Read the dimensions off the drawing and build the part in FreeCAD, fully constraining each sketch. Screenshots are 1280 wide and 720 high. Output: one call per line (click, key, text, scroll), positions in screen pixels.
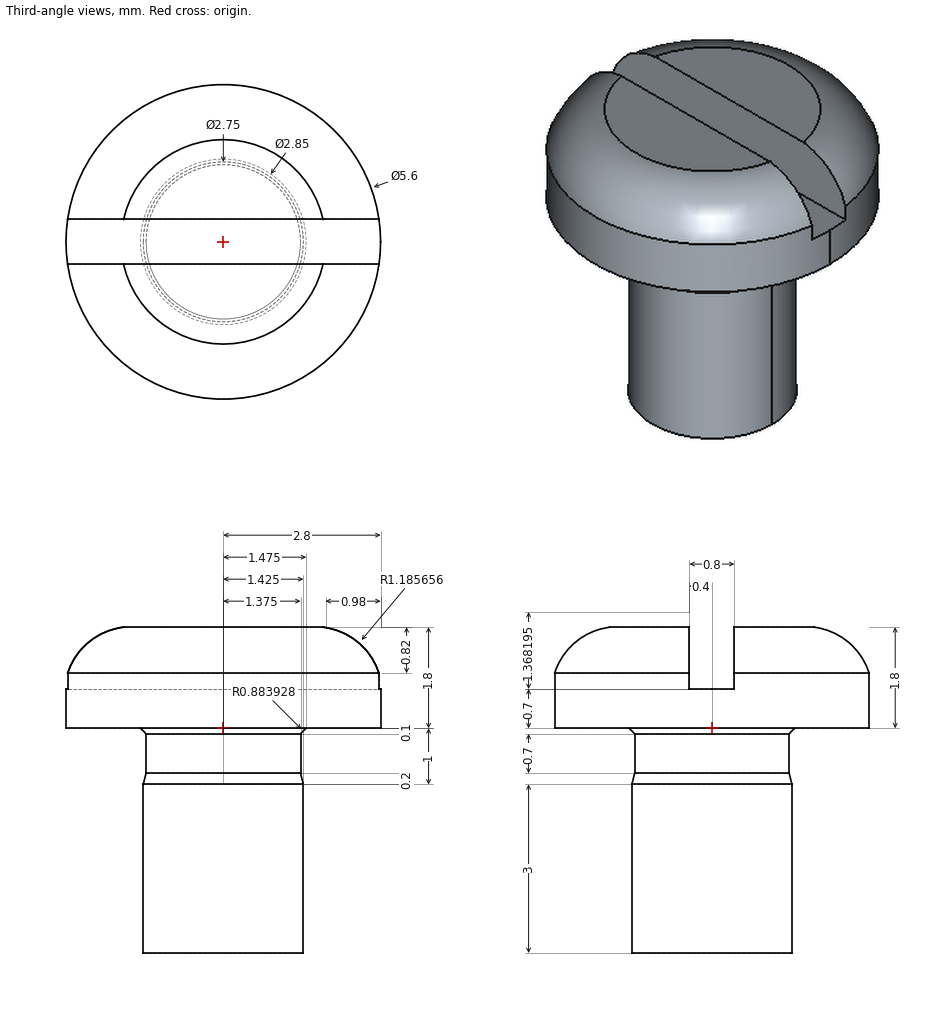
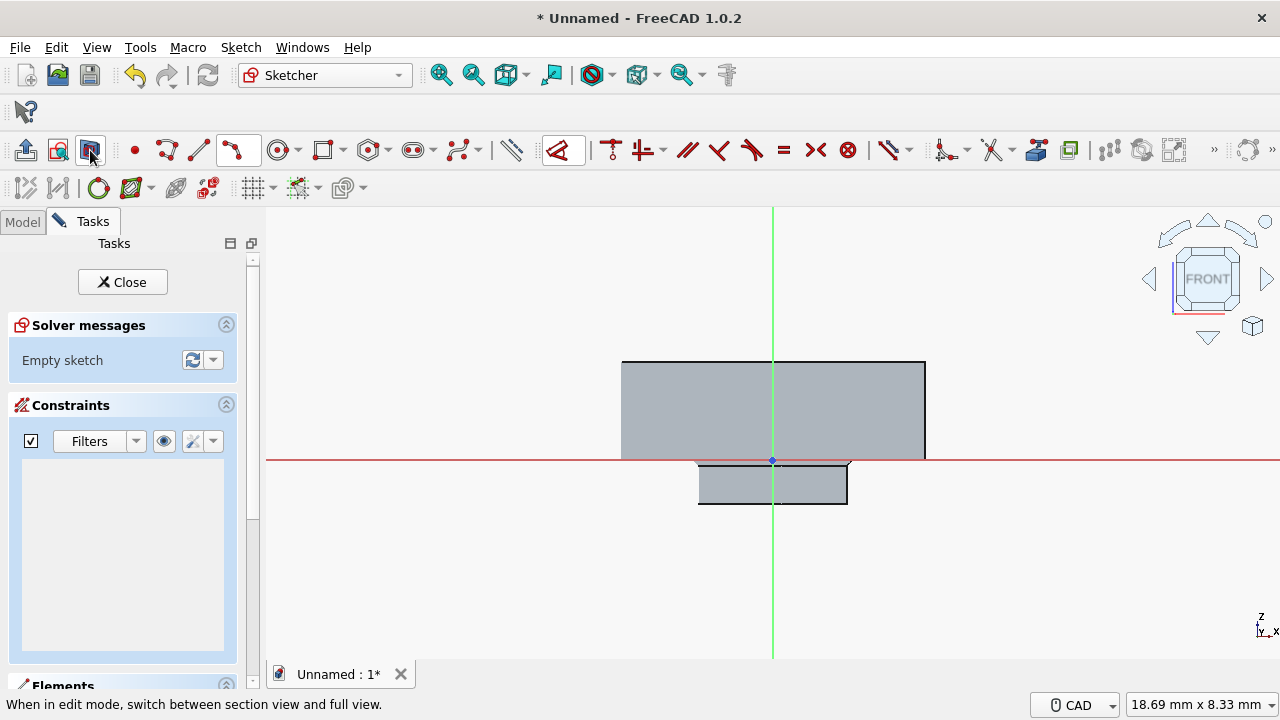
scroll(839, 501, up, 8)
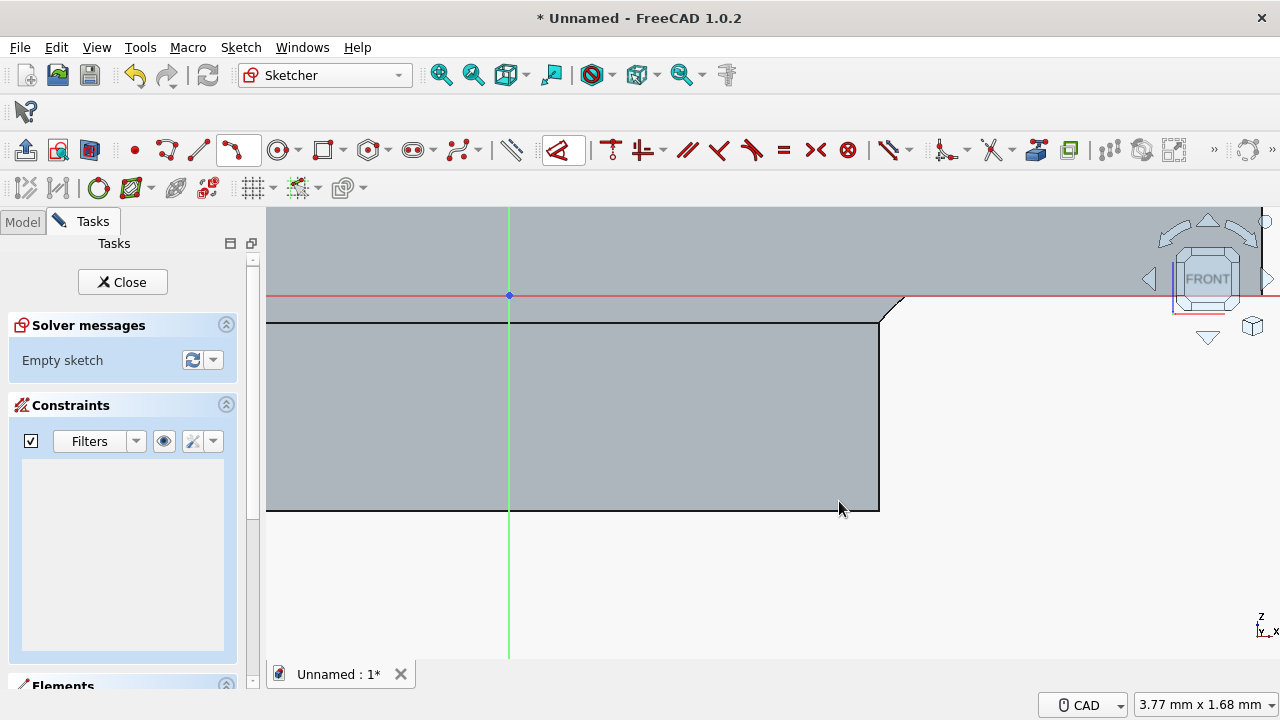
click(168, 150)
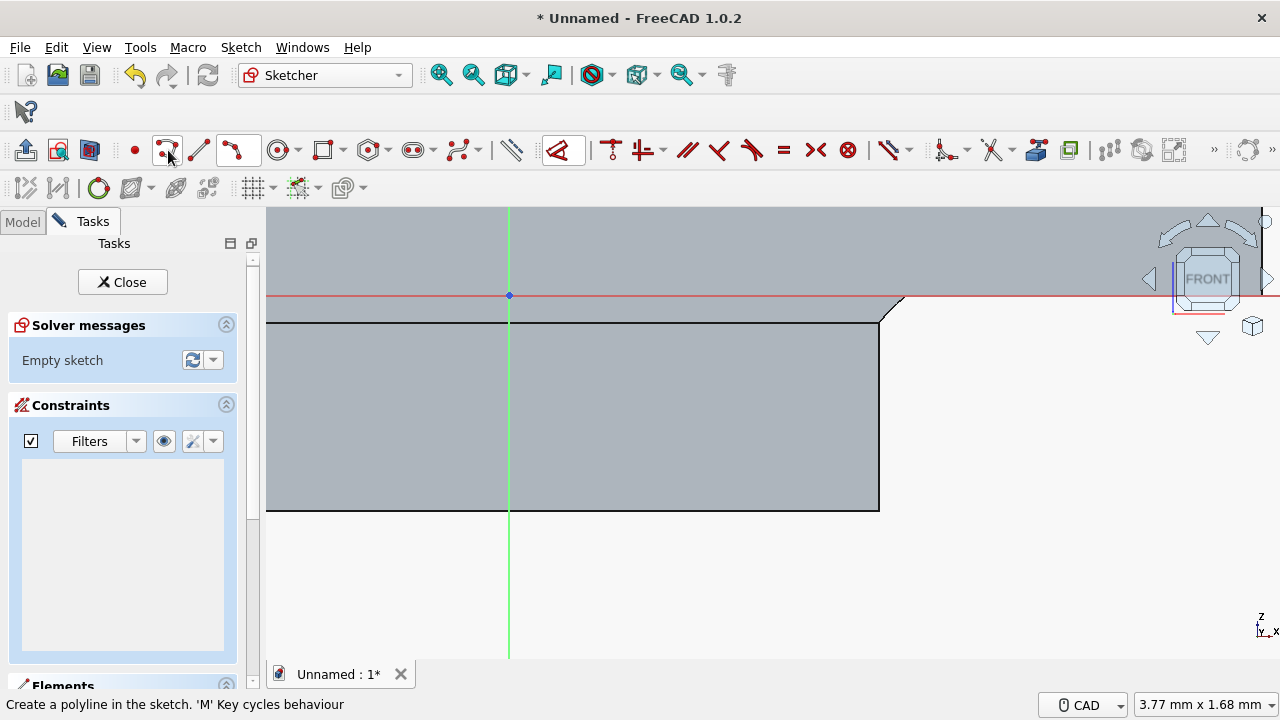
click(509, 511)
click(879, 511)
click(892, 565)
click(518, 565)
click(509, 512)
key(Escape)
key(Escape)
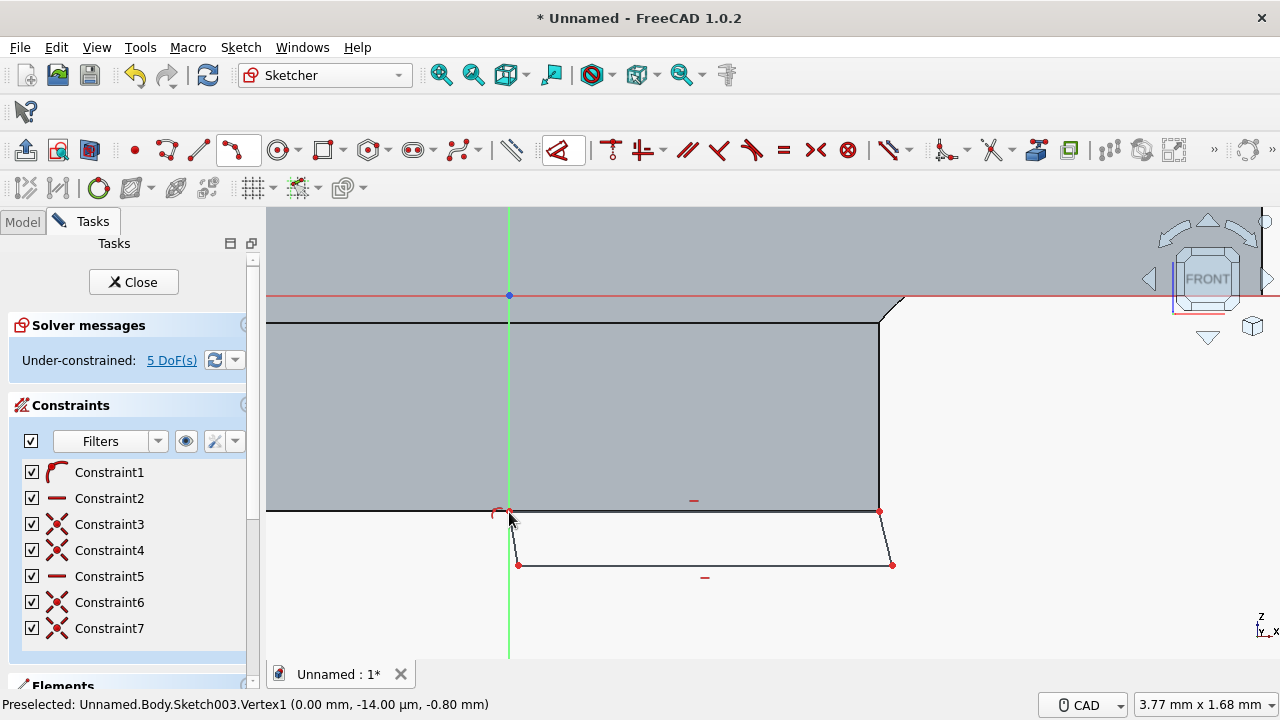
click(512, 528)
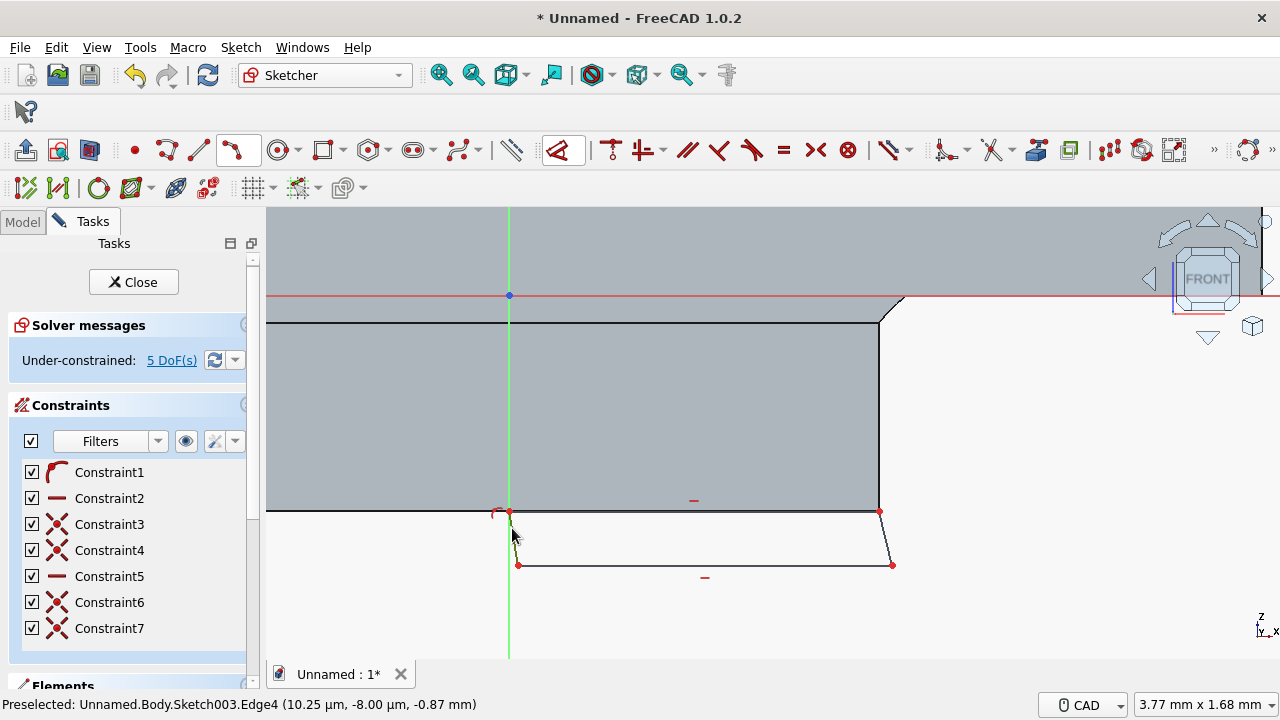
click(666, 150)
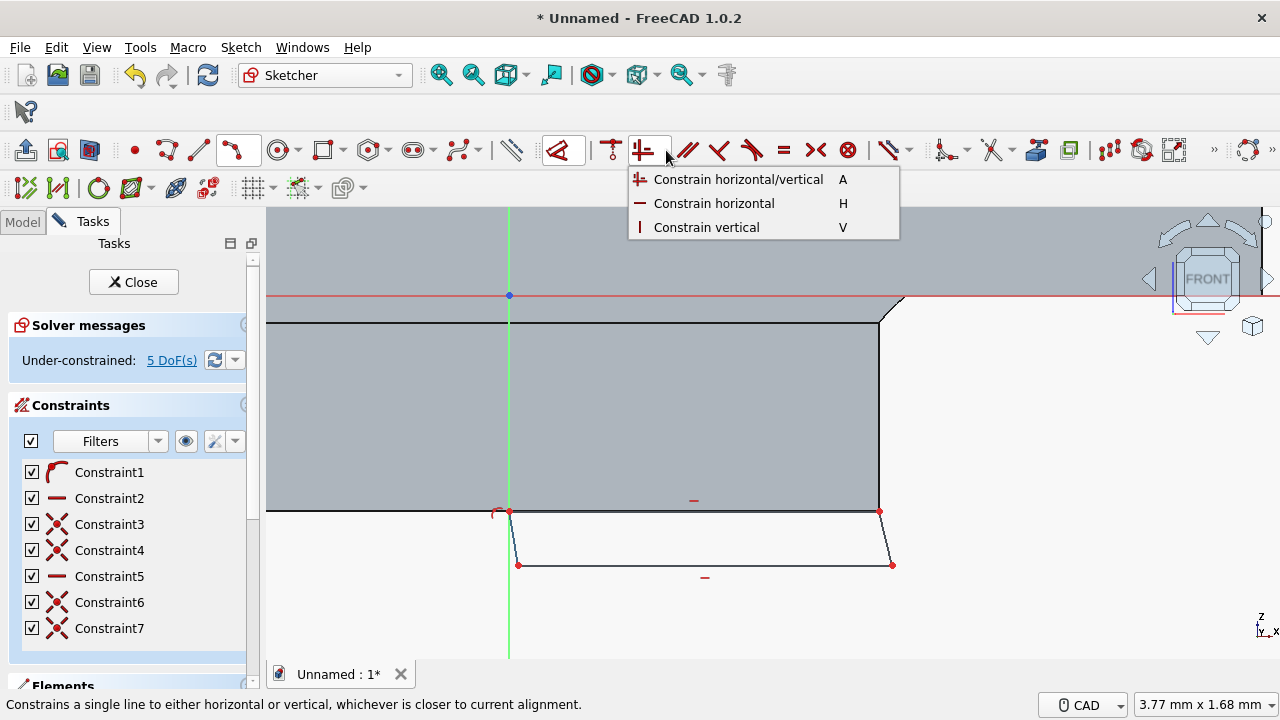
click(764, 227)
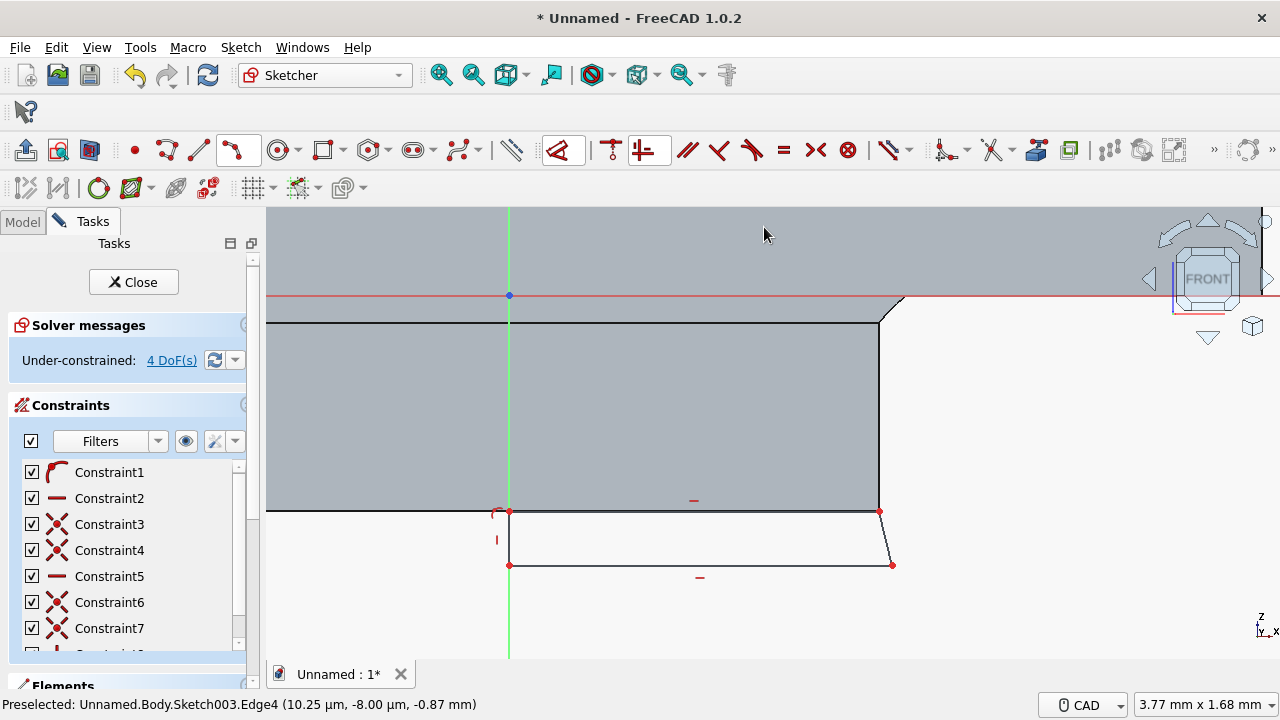
click(892, 566)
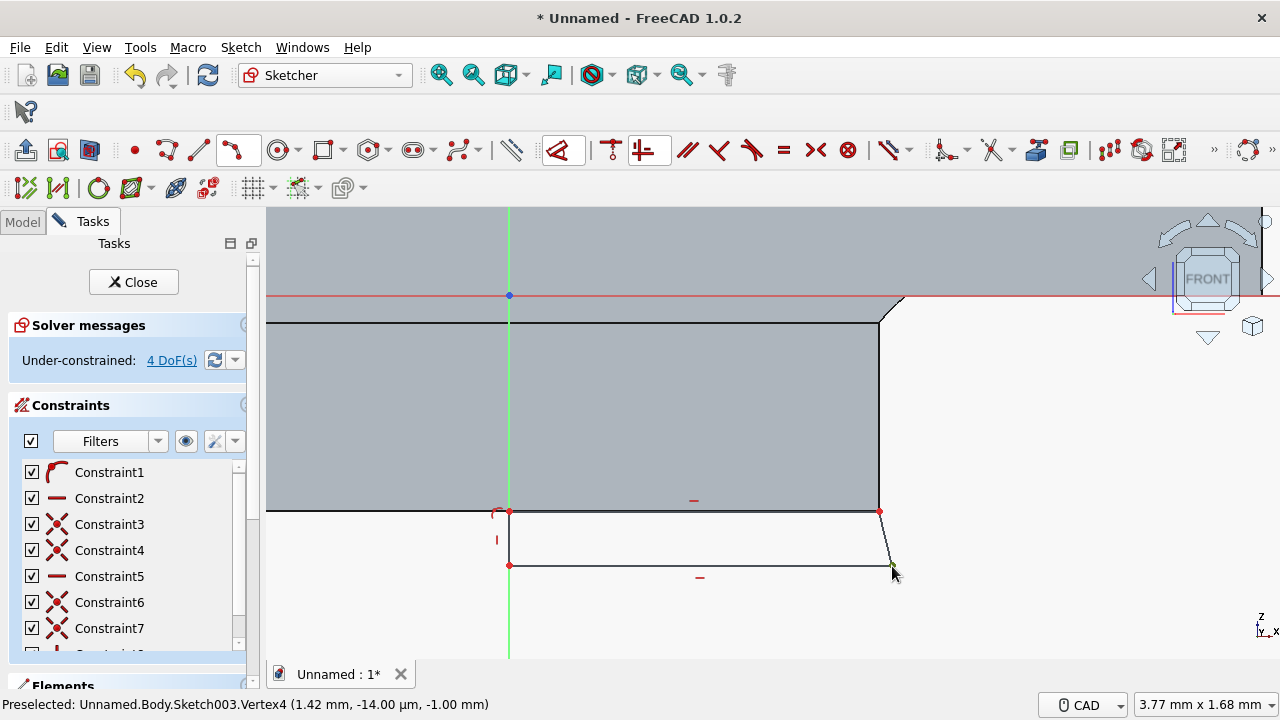
click(580, 150)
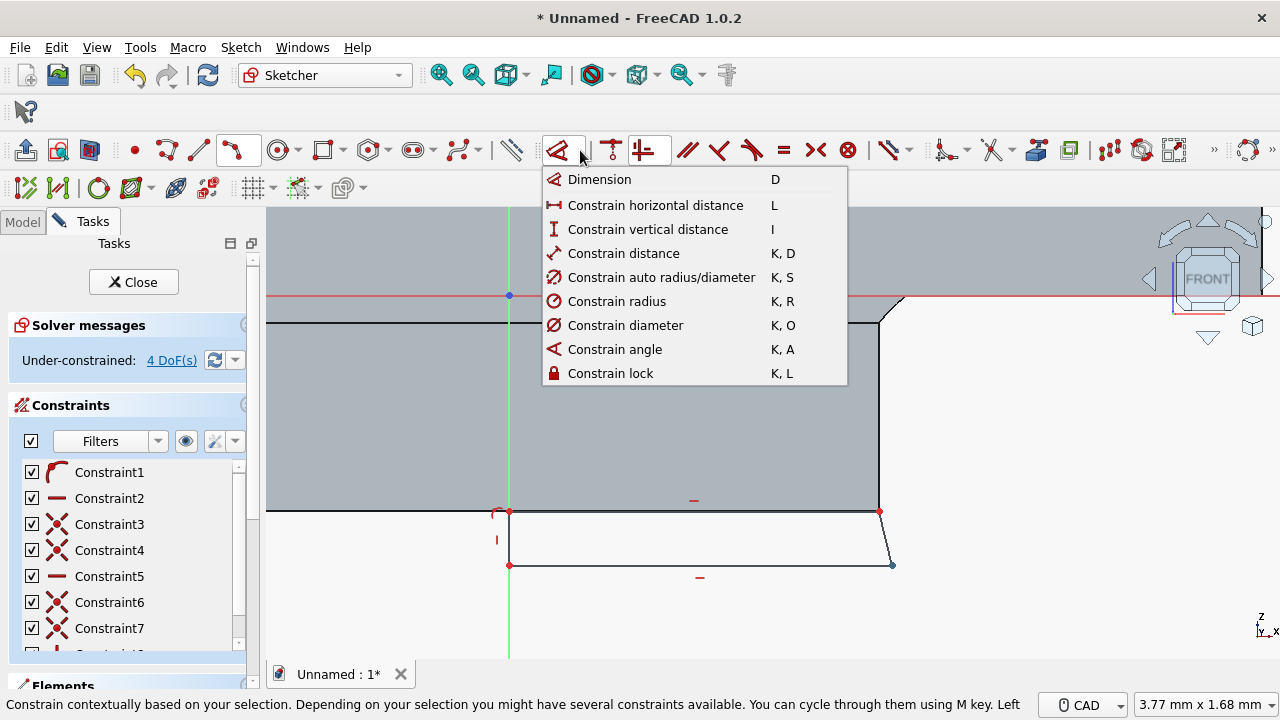
click(695, 229)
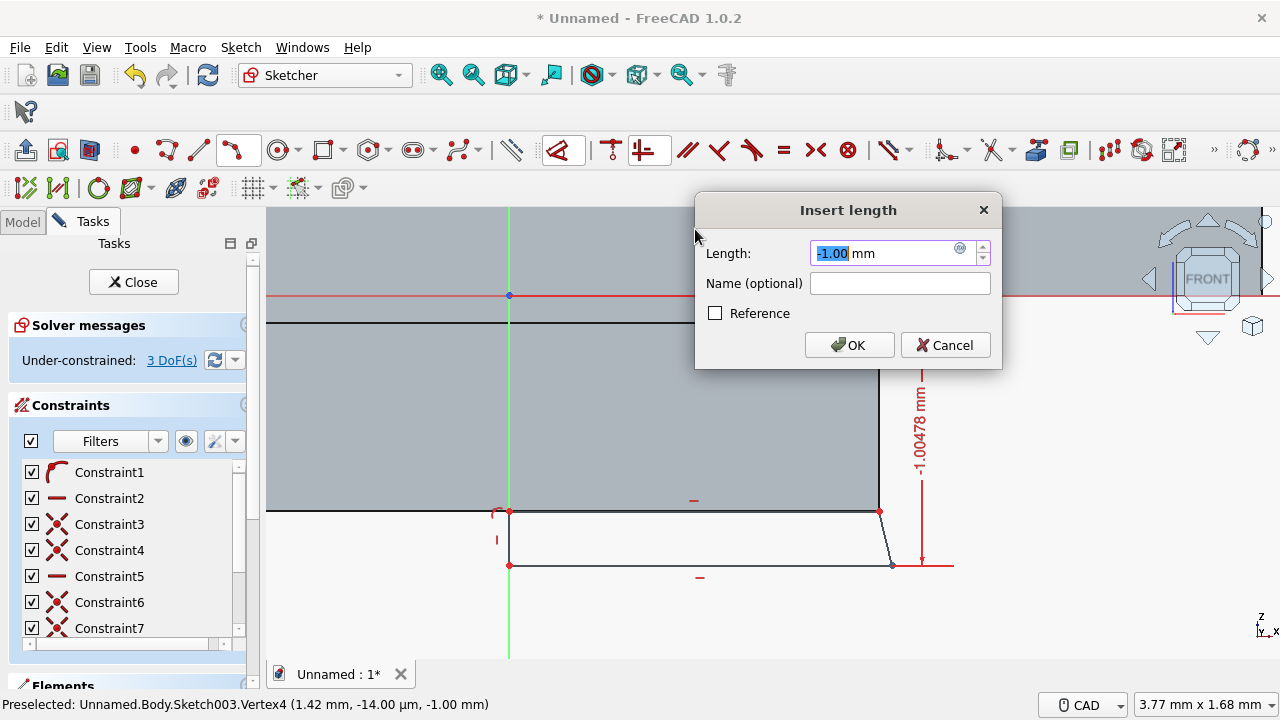
text(-1)
key(Return)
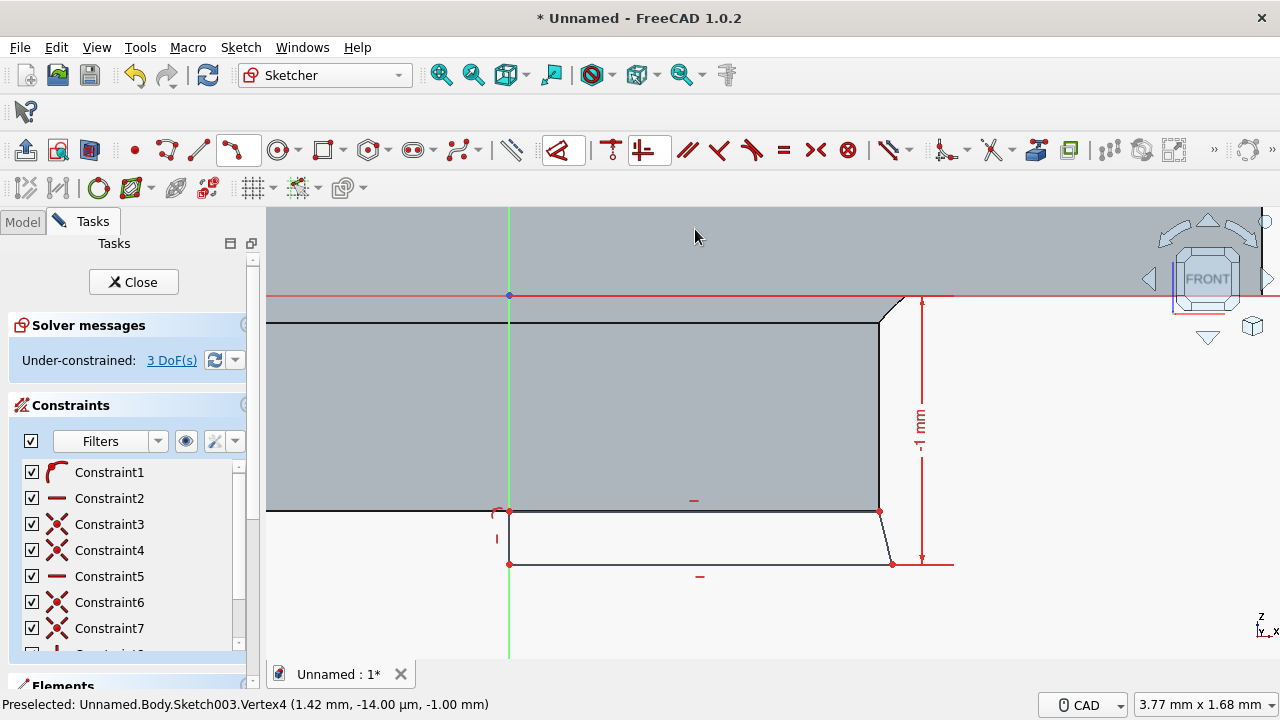
click(509, 549)